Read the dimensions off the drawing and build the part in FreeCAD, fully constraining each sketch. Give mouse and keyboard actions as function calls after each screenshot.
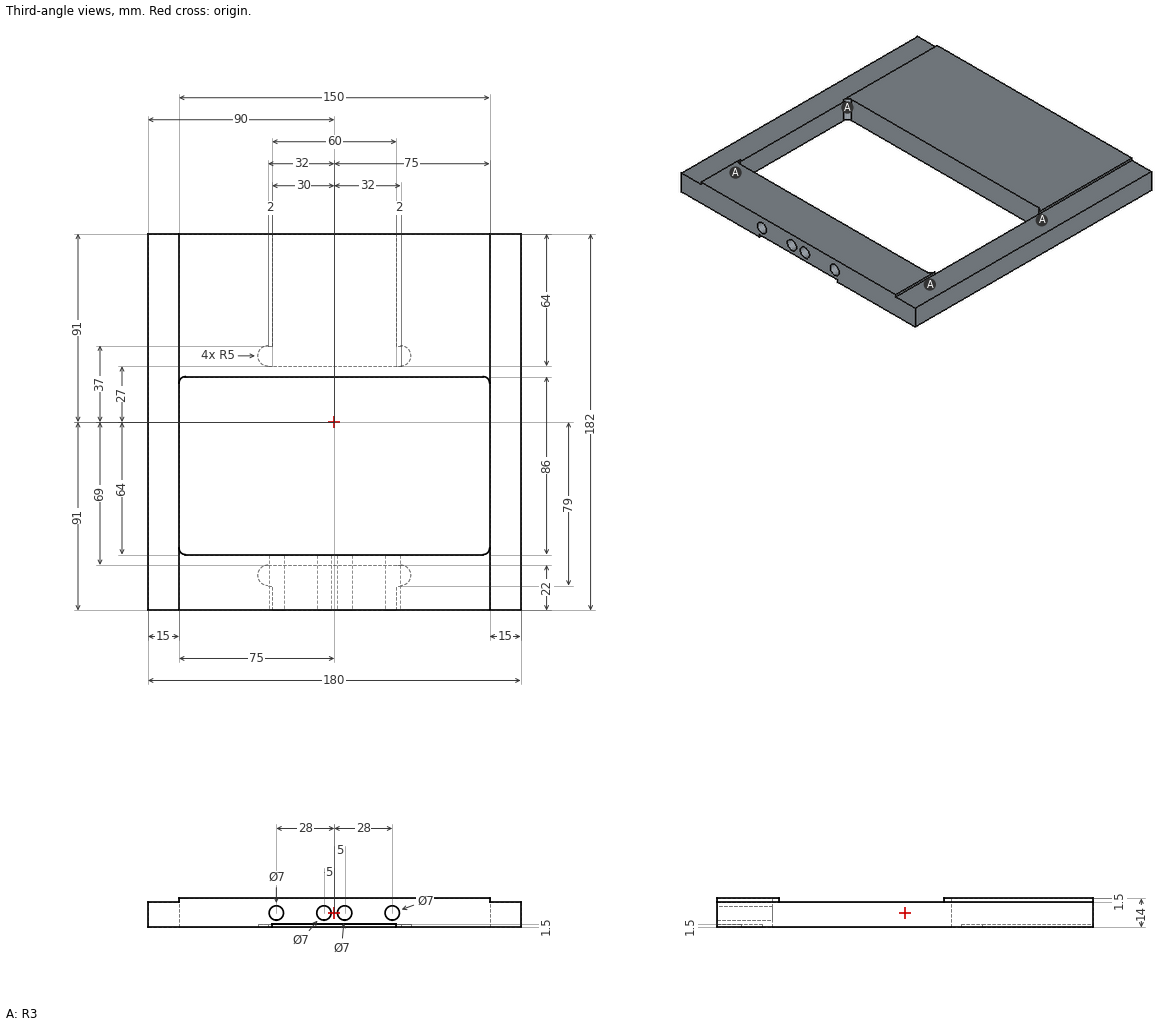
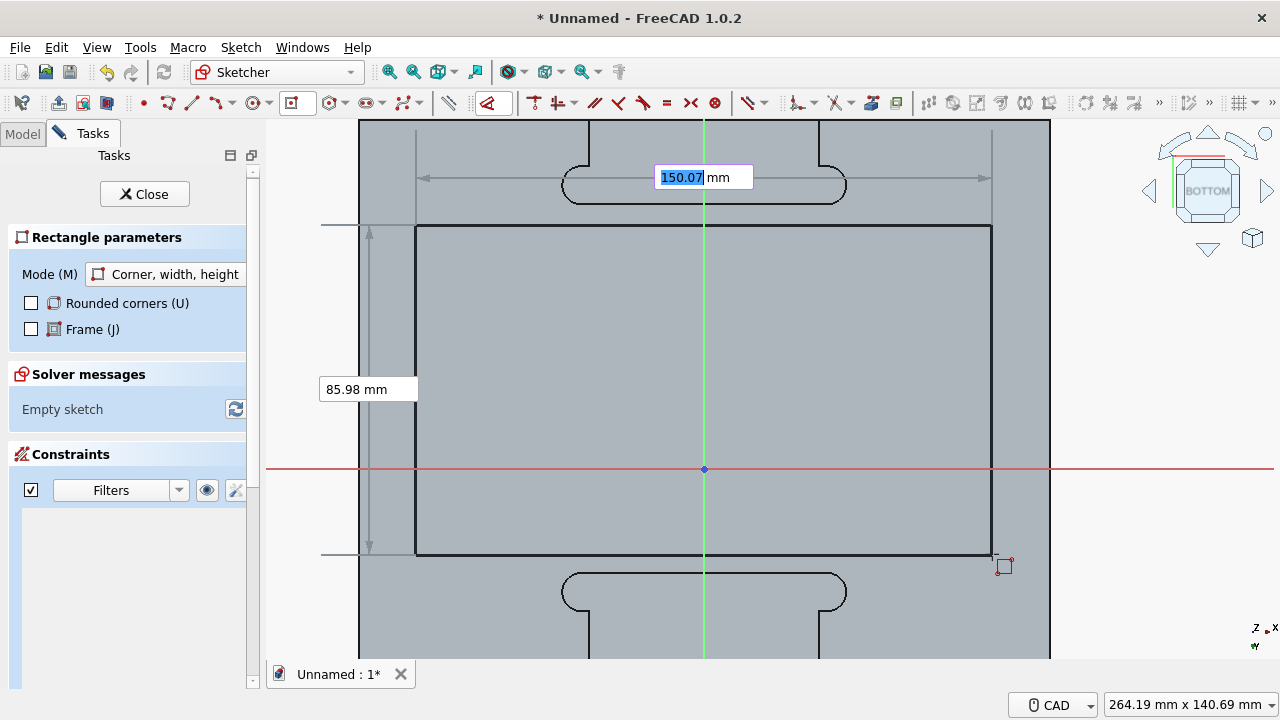
text(150)
key(Tab)
text(86)
key(Return)
key(Escape)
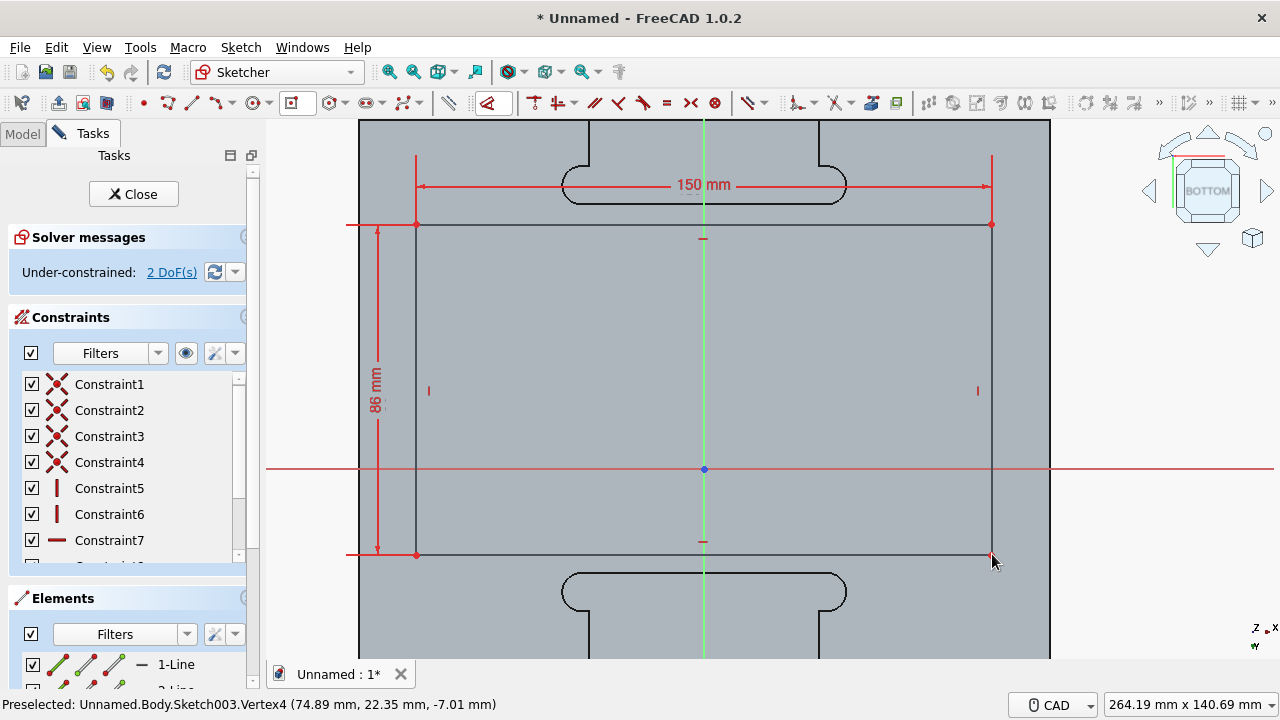
click(416, 225)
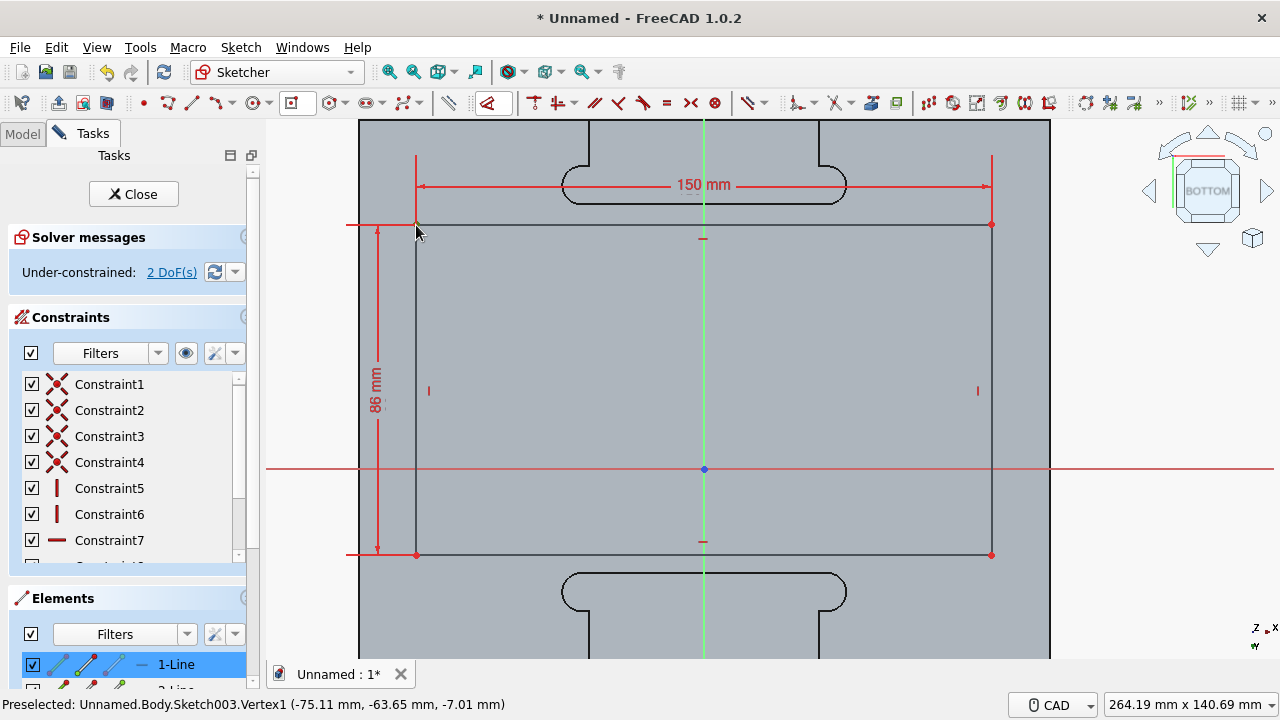
key(l)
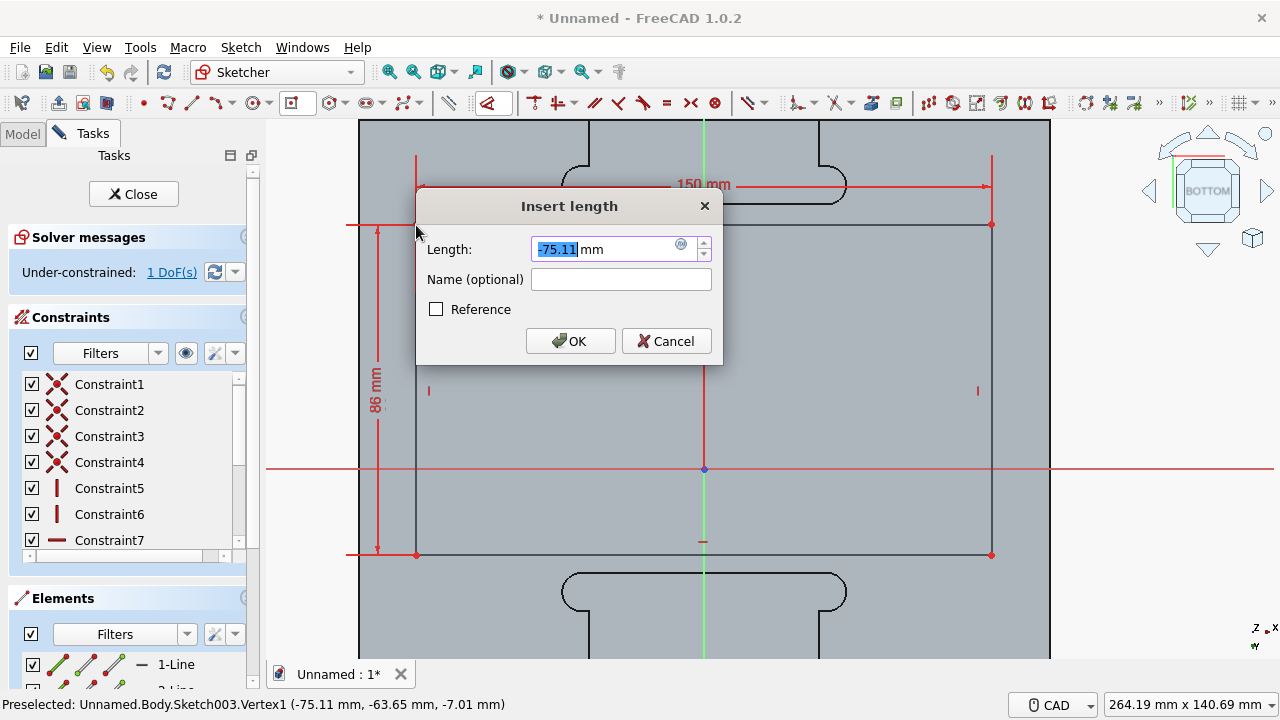
text(-75)
key(Return)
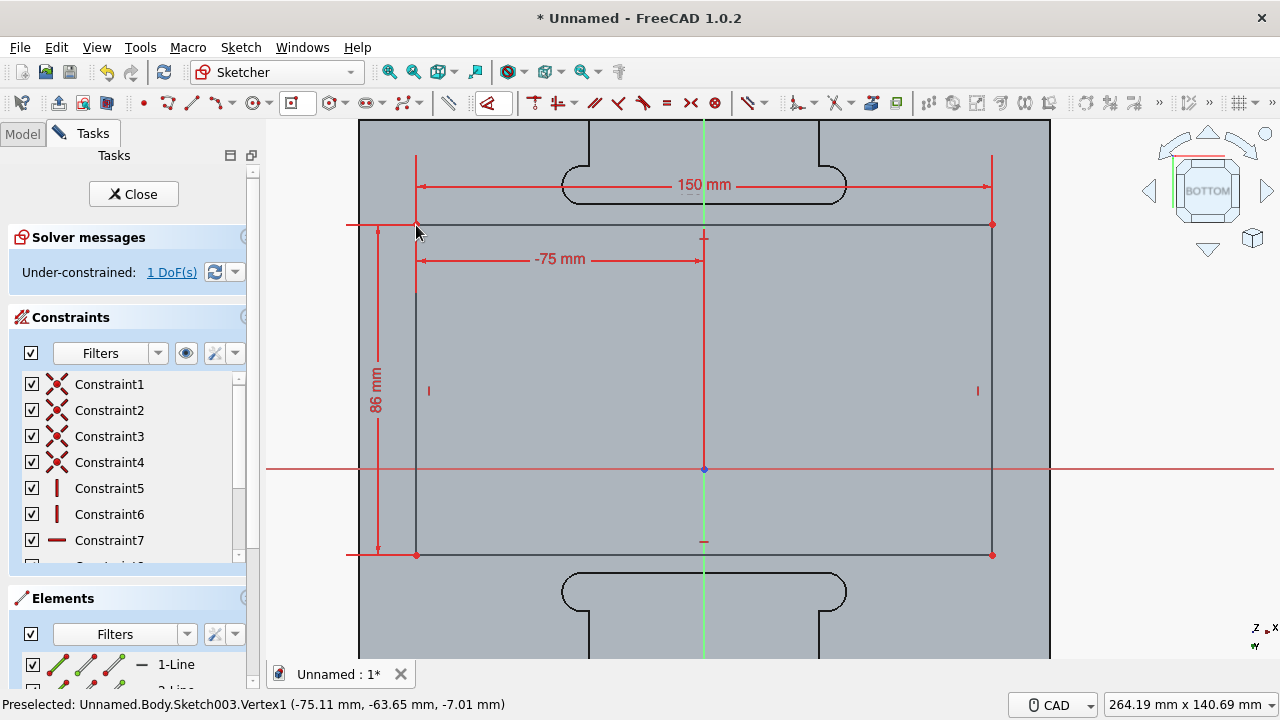
click(416, 225)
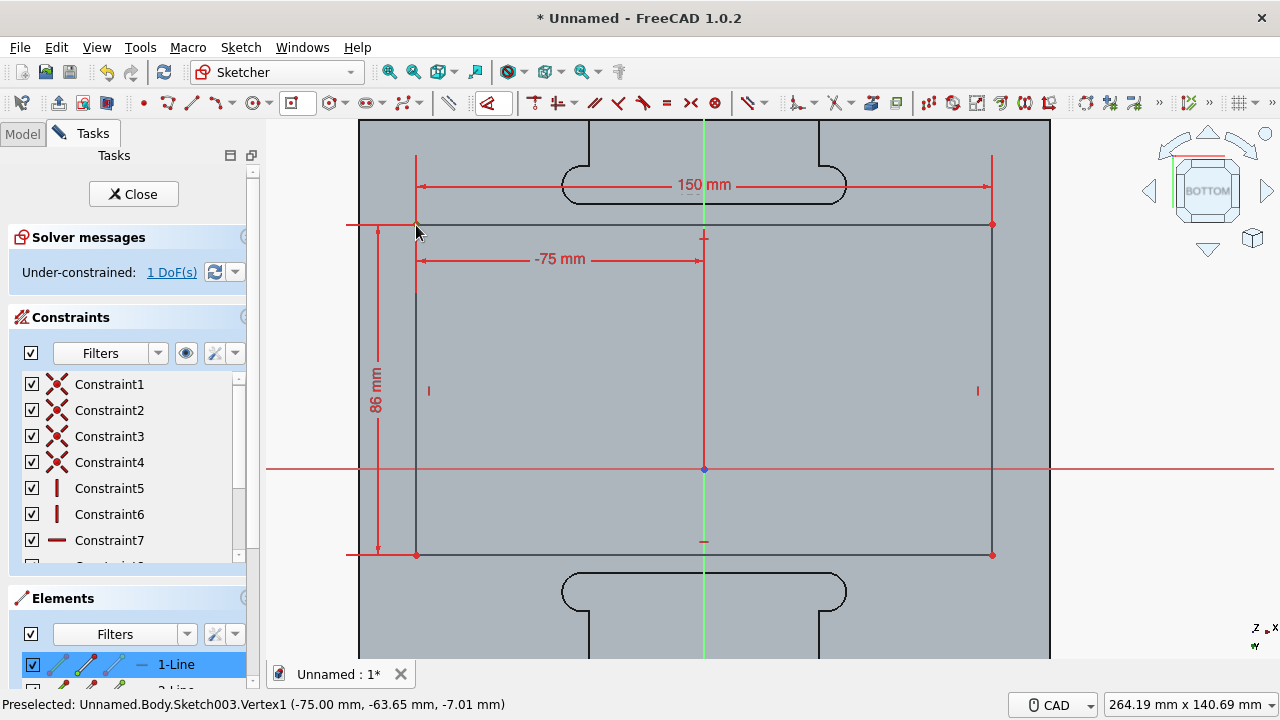
click(506, 104)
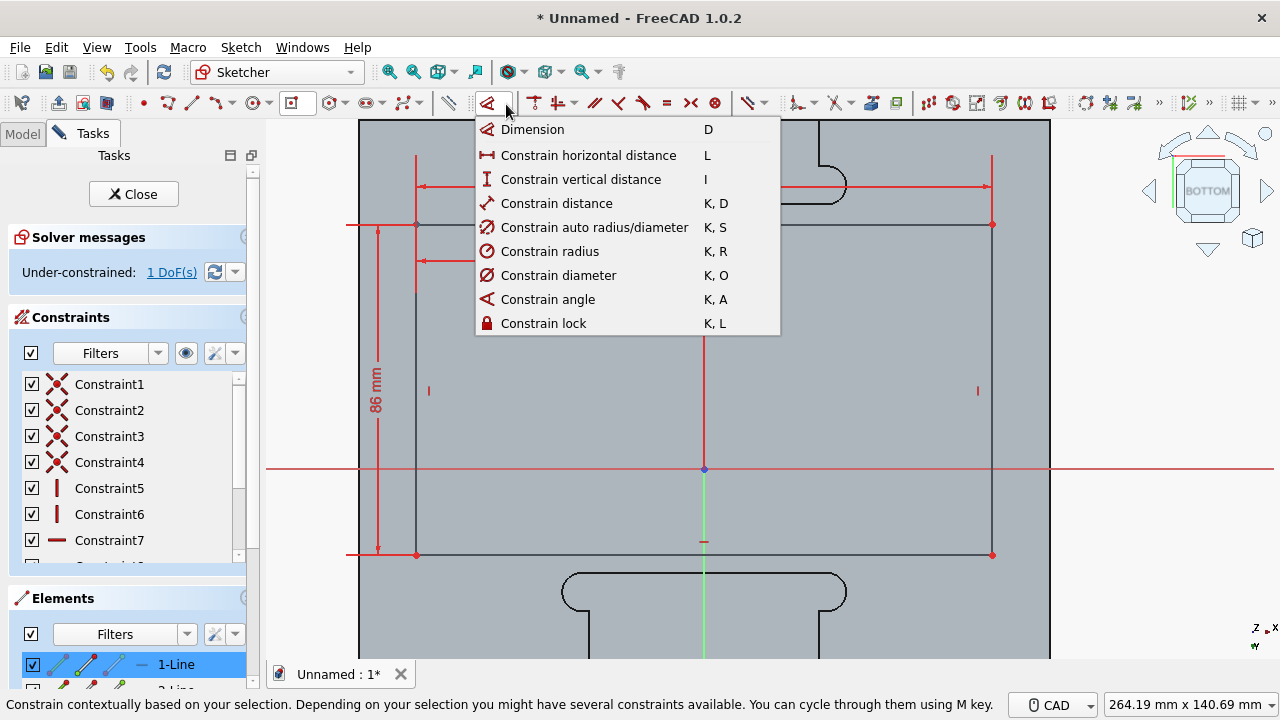
click(628, 179)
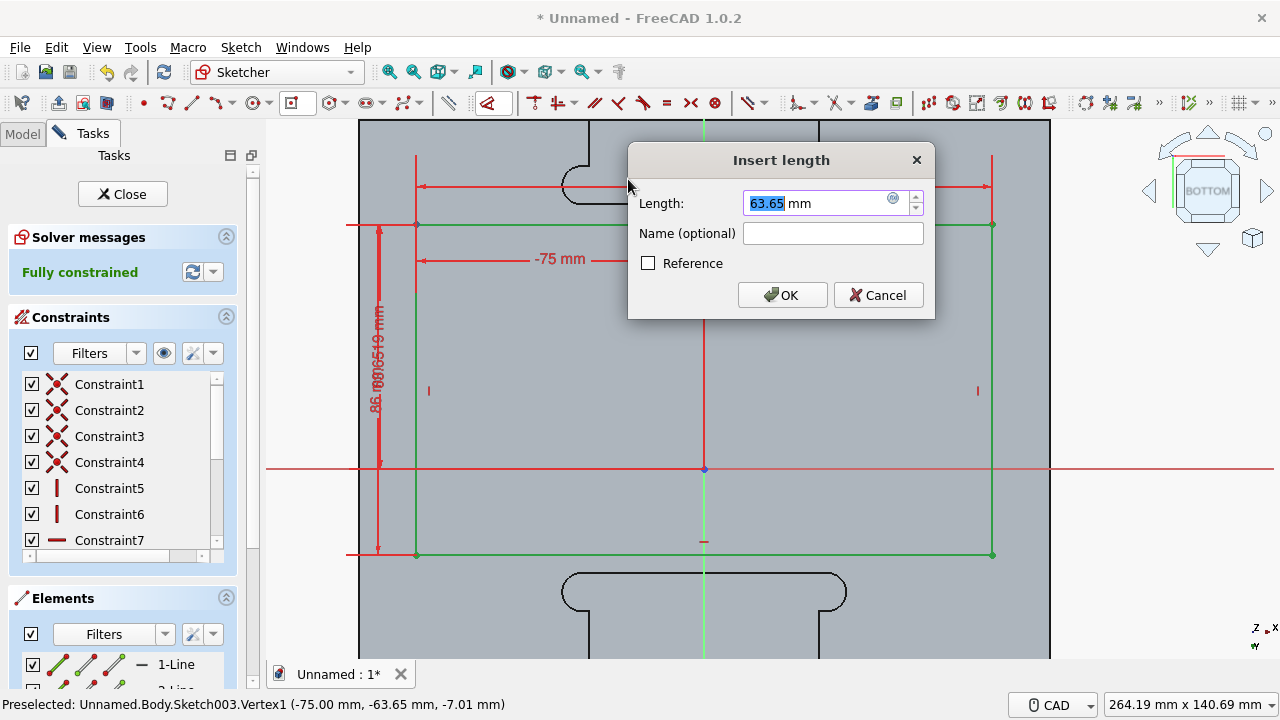
text(64)
key(Return)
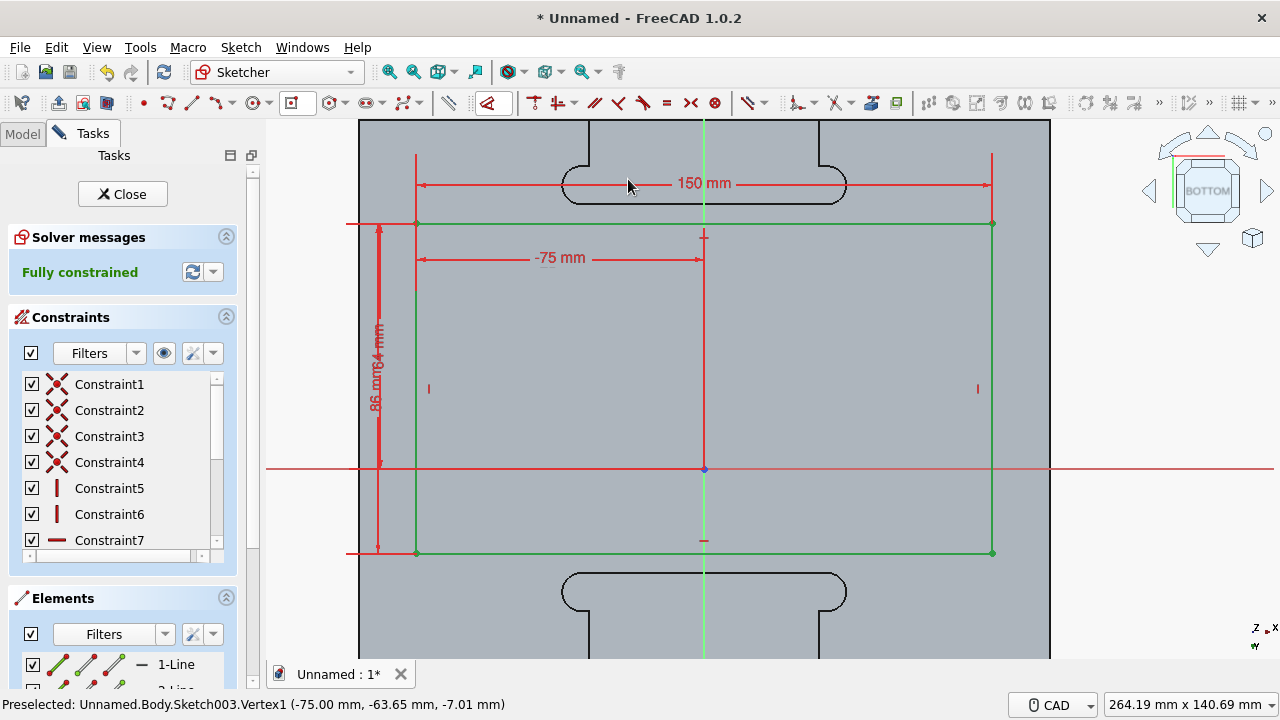
click(123, 194)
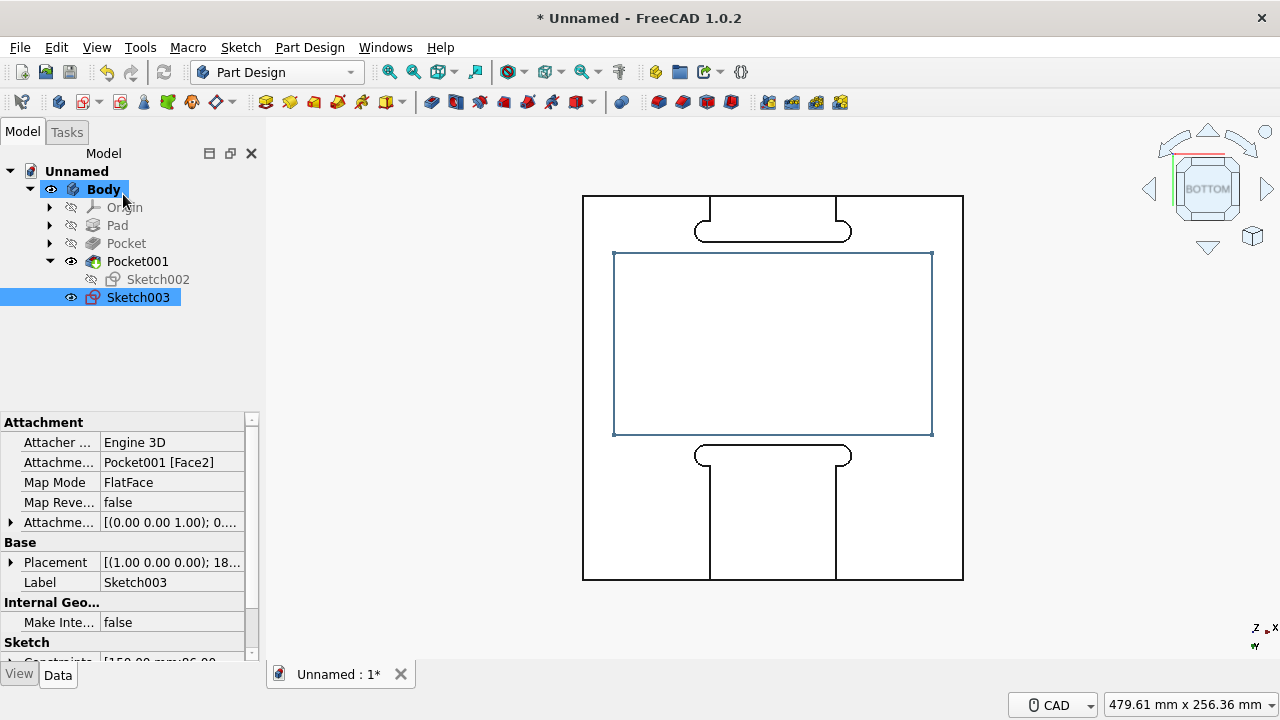
click(432, 102)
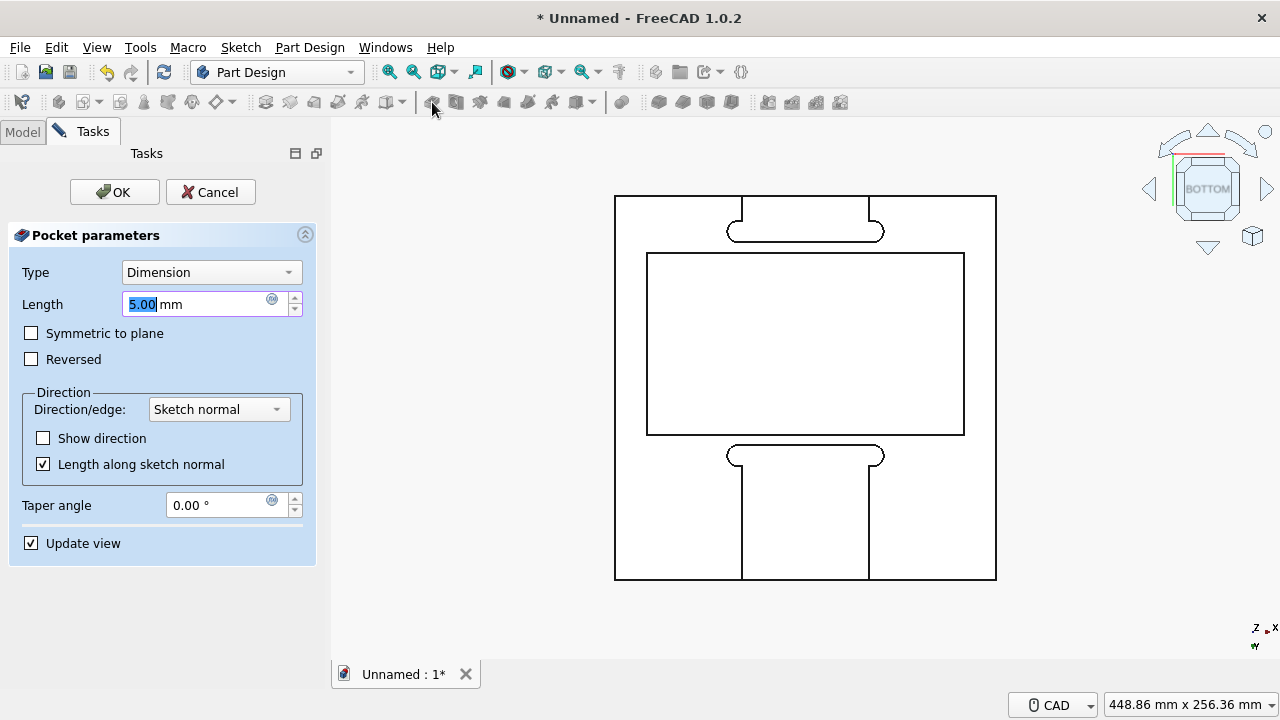
click(212, 272)